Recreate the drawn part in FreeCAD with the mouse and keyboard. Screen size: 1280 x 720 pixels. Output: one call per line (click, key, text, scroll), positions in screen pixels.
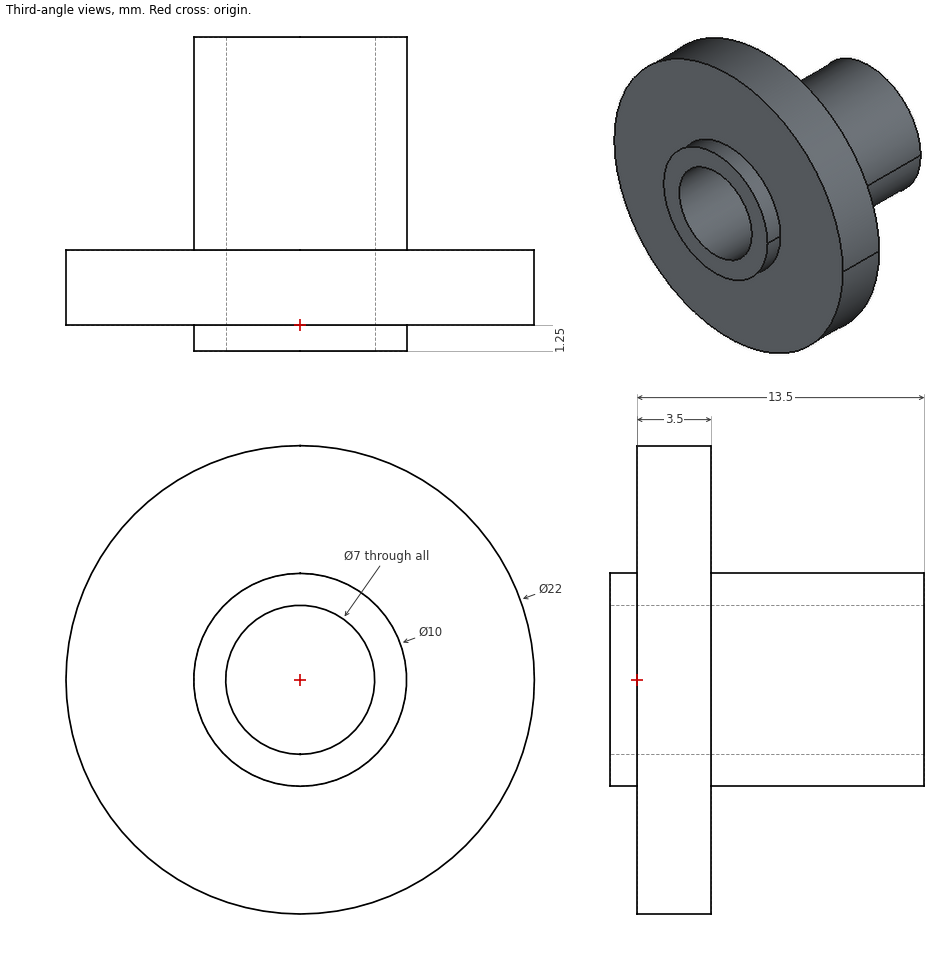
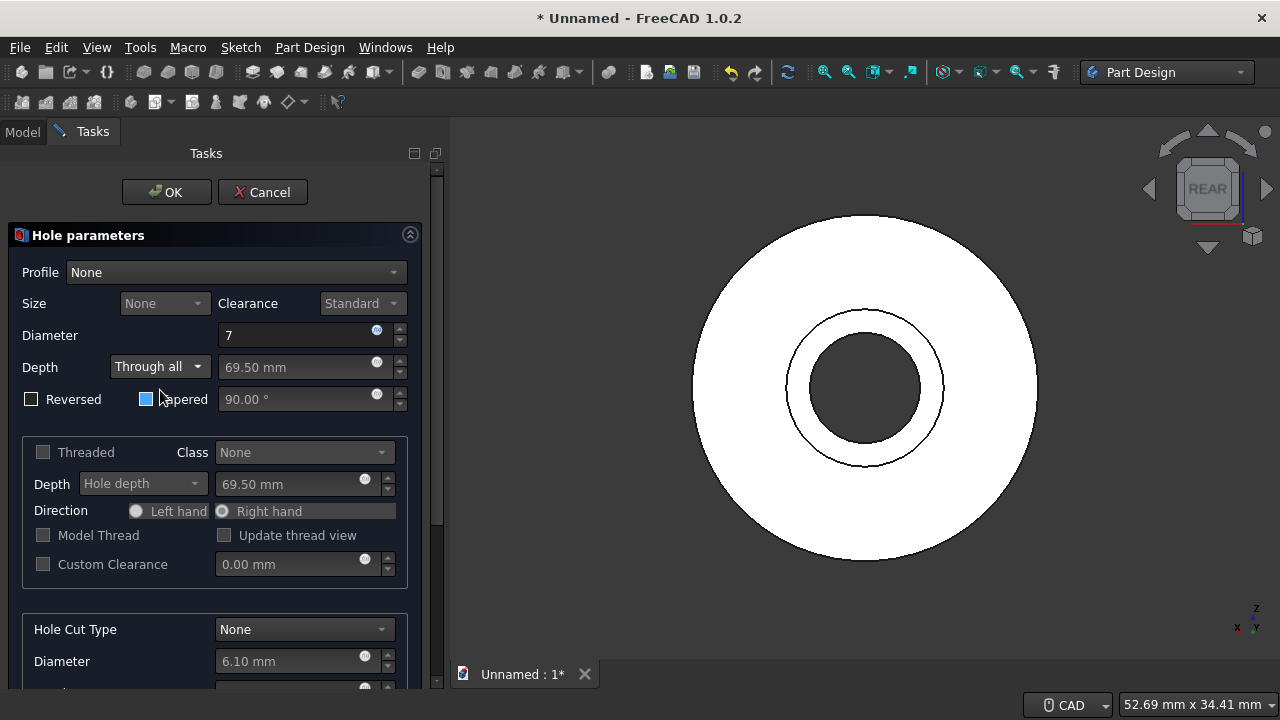
click(167, 192)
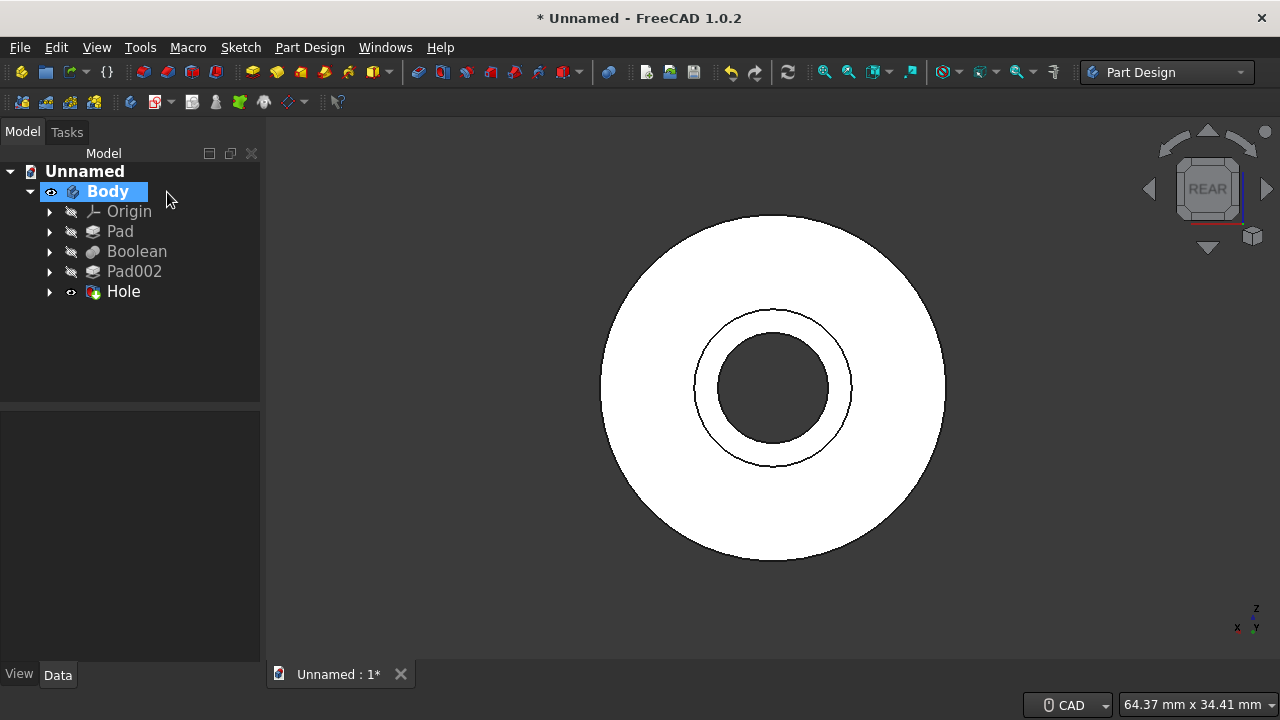
key(0)